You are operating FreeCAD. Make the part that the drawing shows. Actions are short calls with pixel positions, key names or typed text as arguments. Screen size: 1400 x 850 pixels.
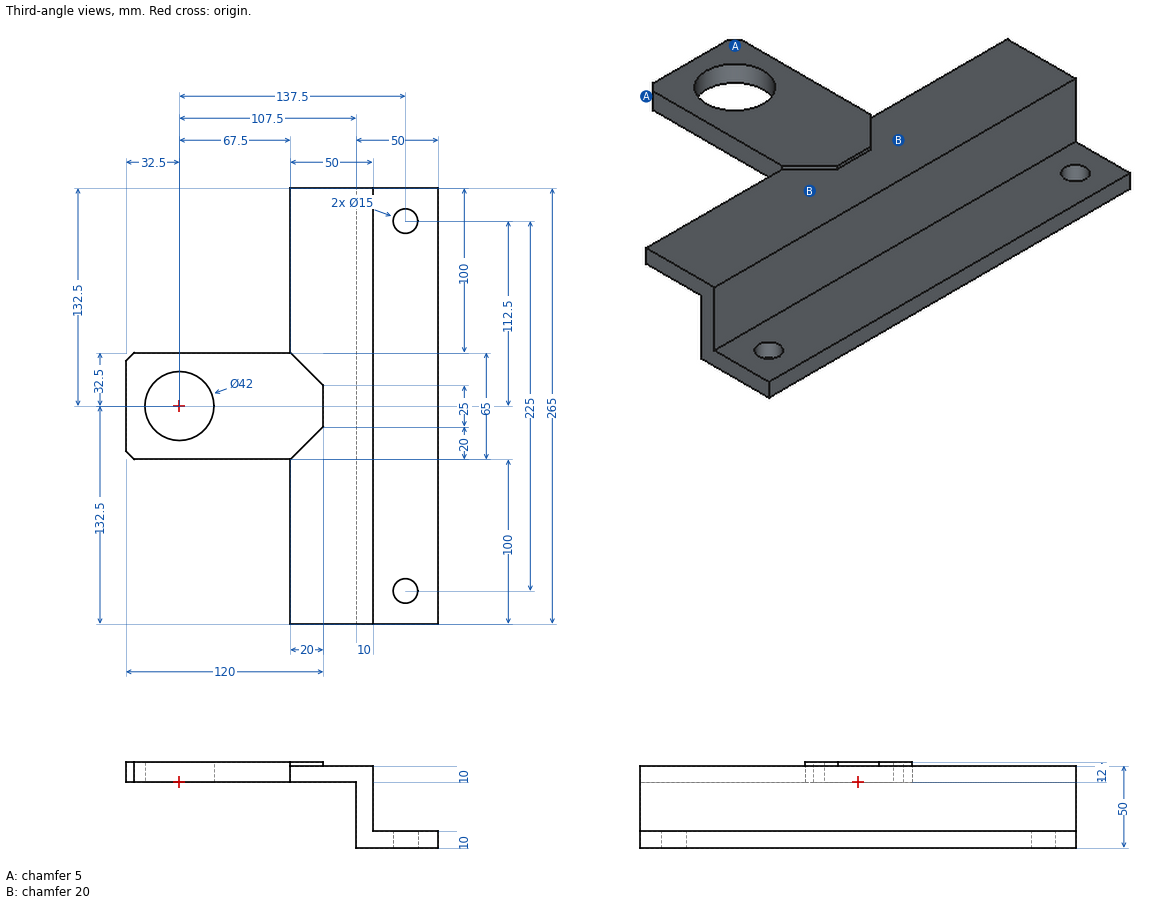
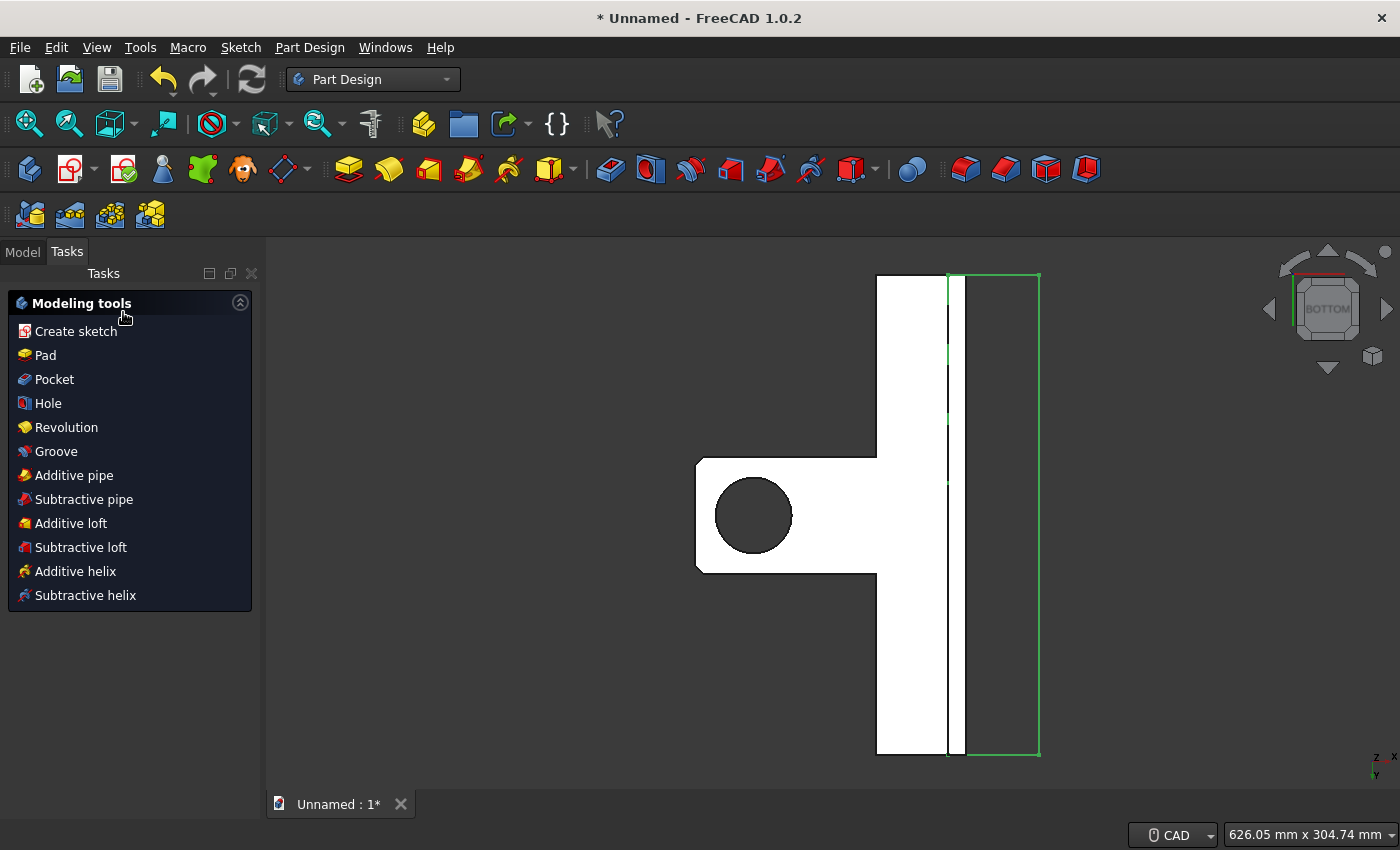
click(350, 170)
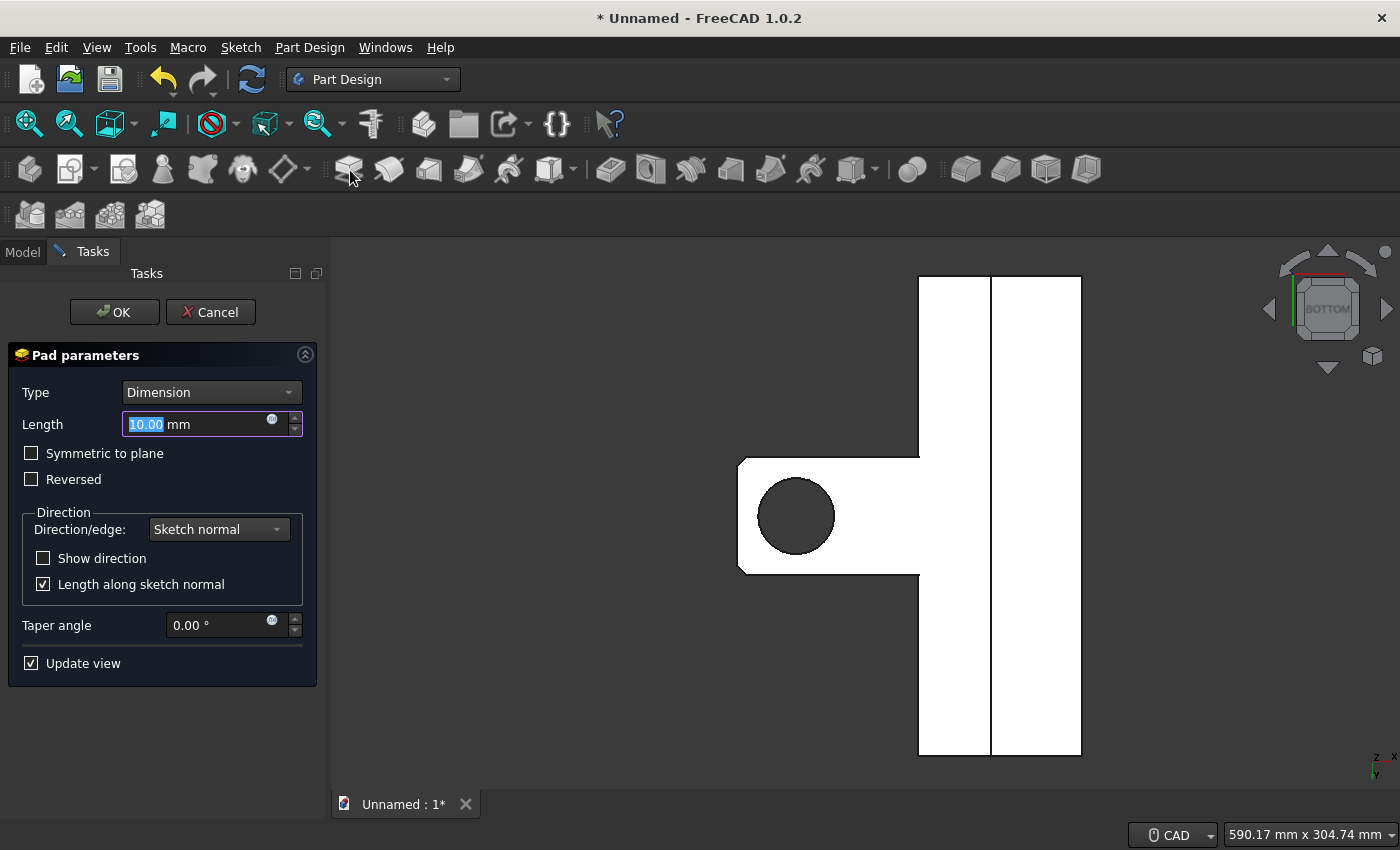
text(10)
key(Tab)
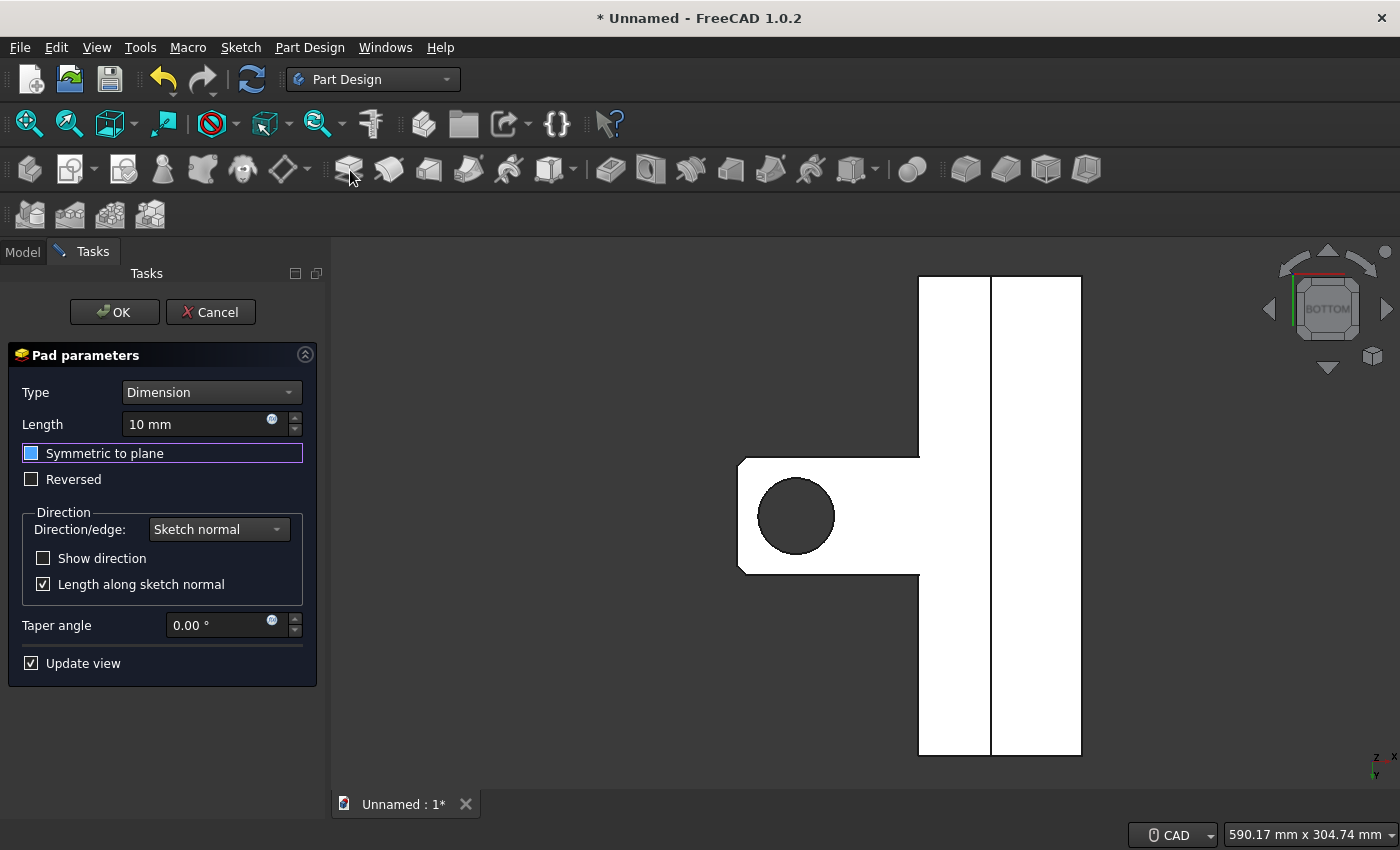
click(30, 479)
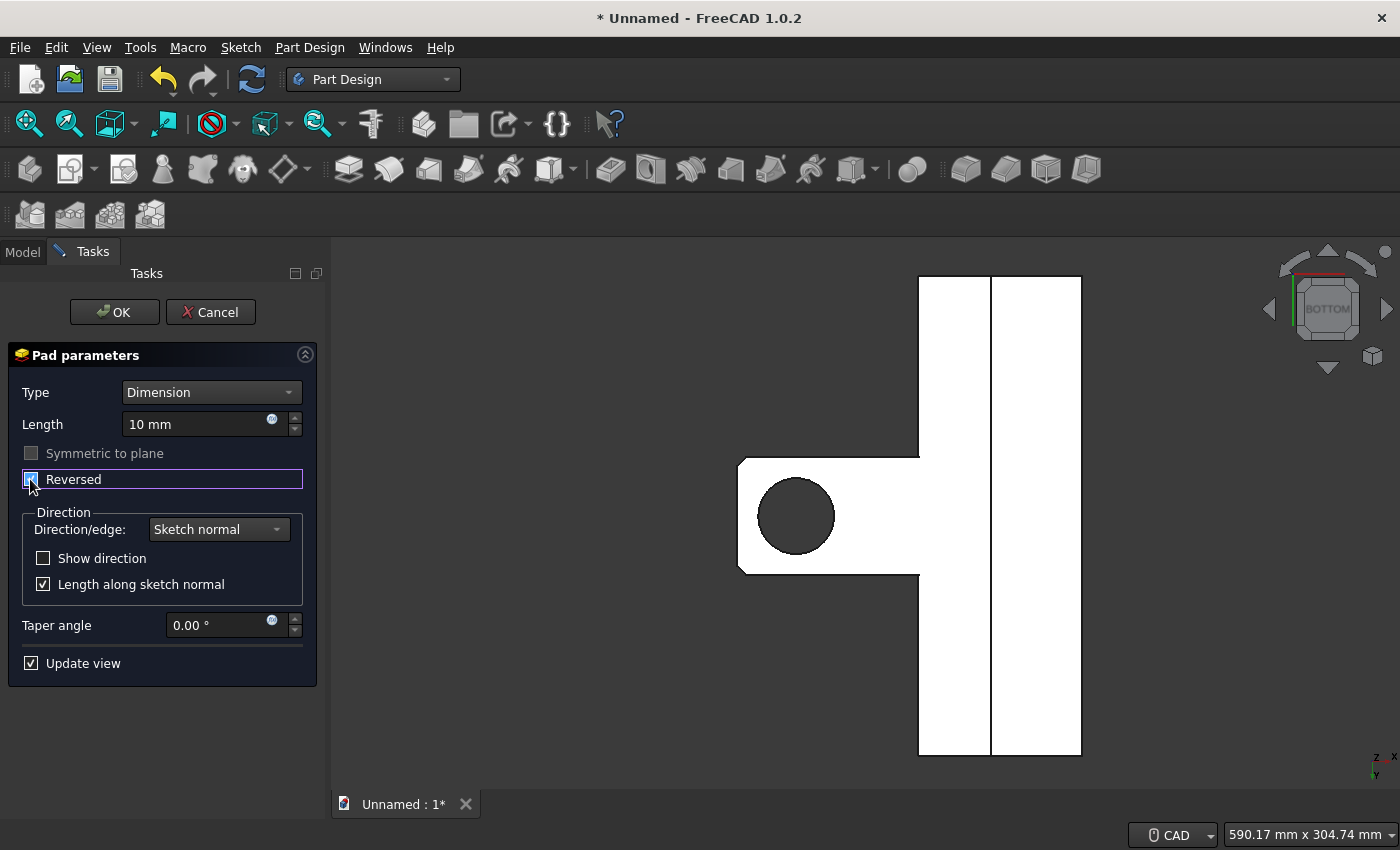
click(115, 312)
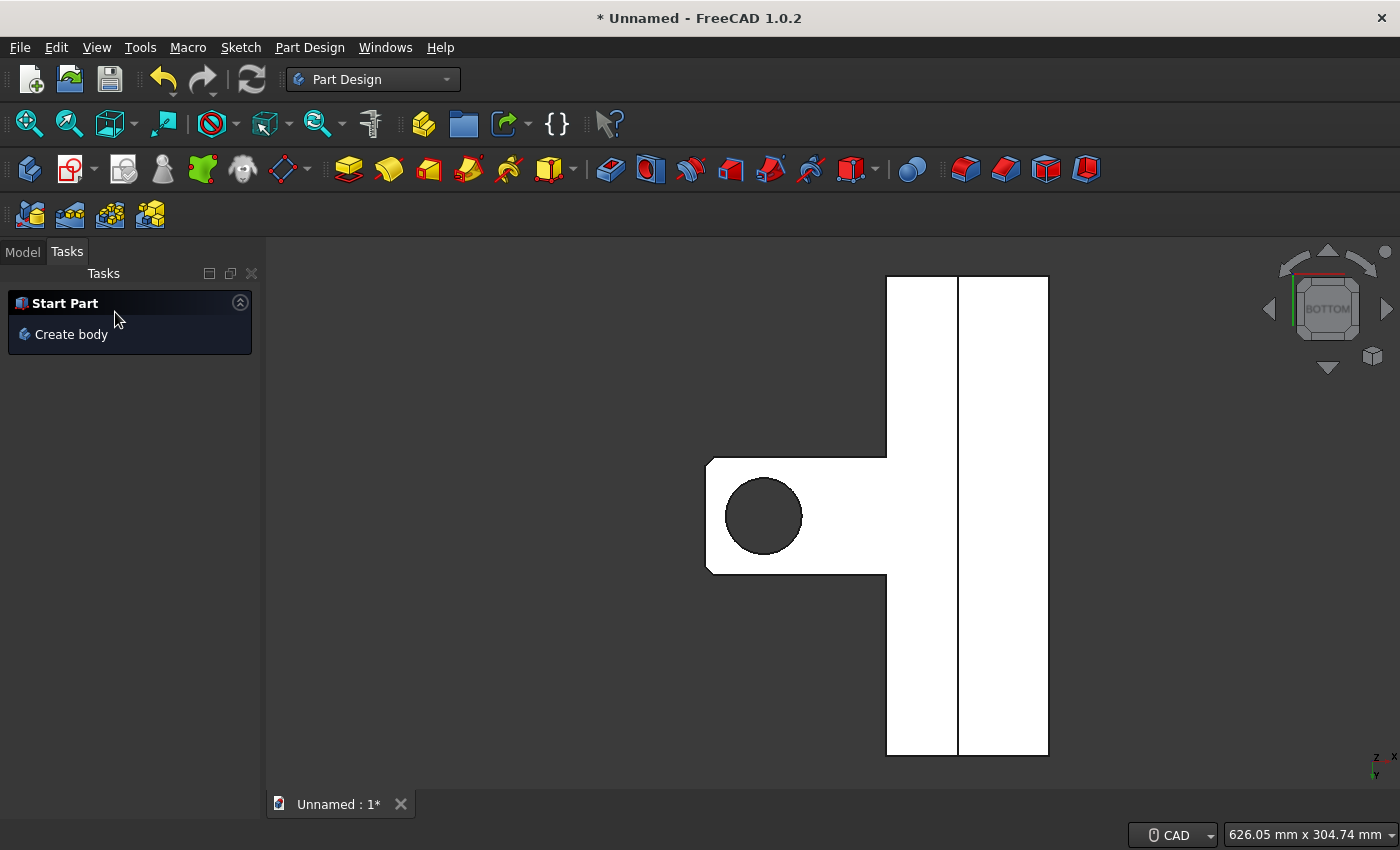
key(0)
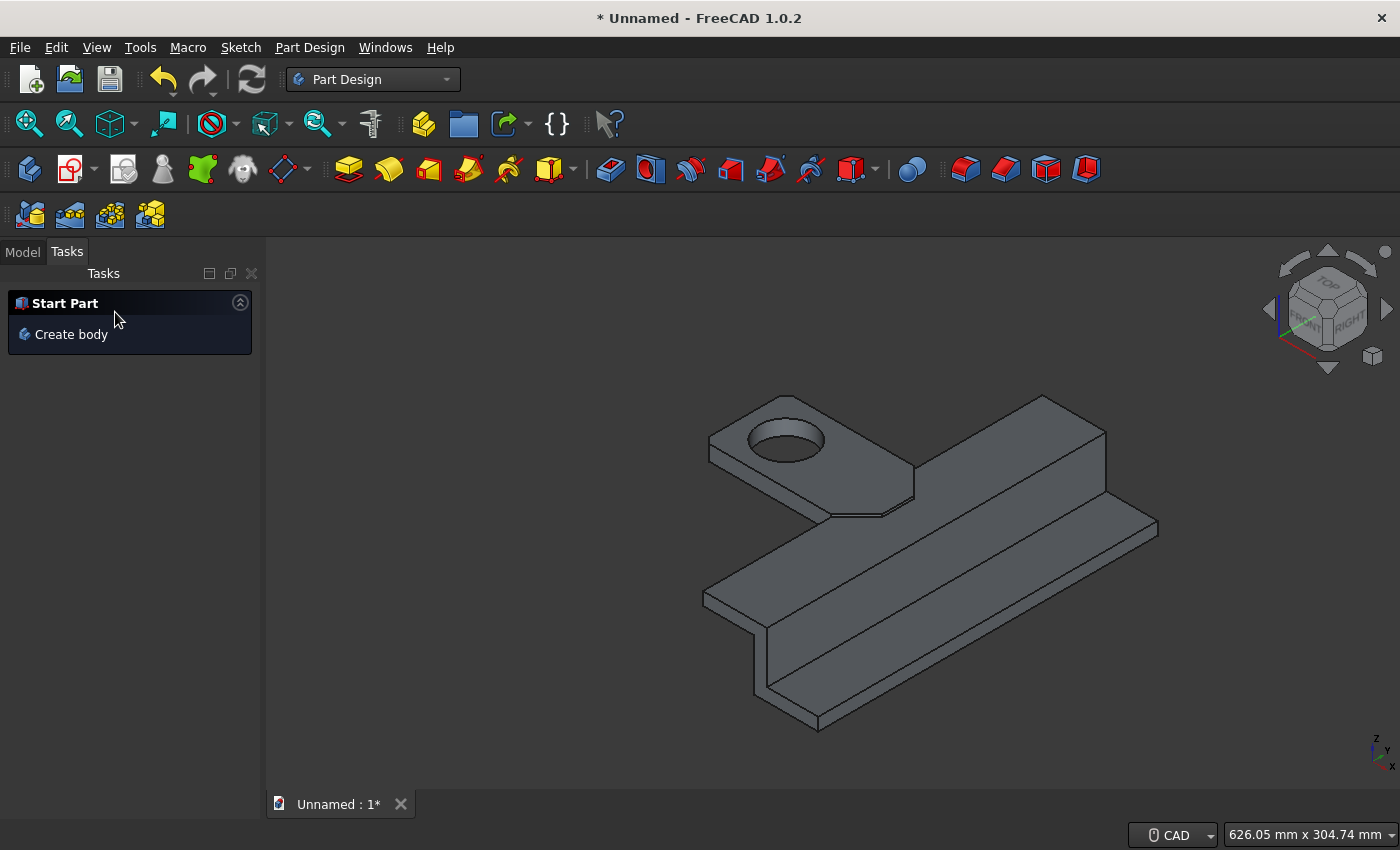
click(1059, 547)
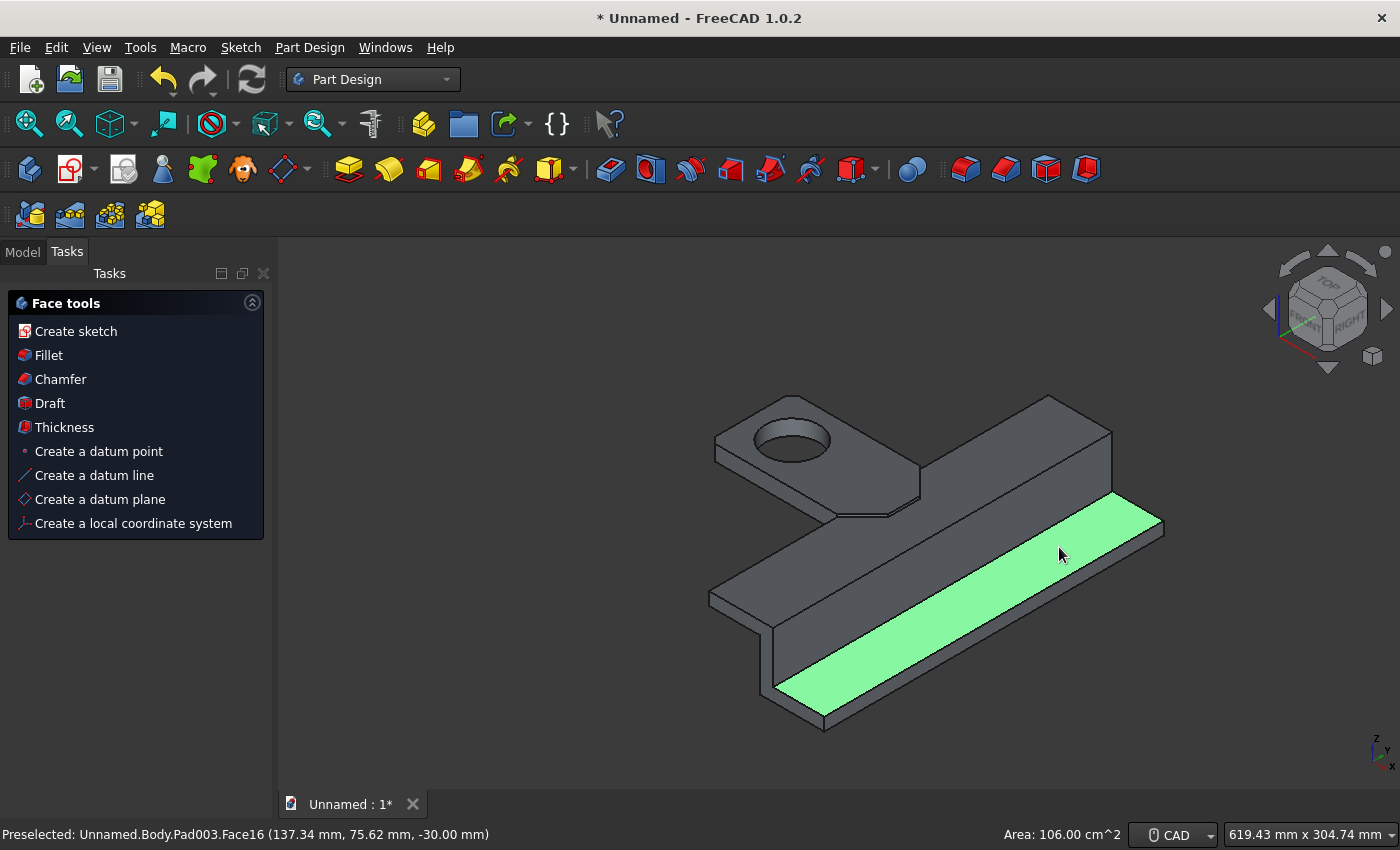
click(70, 170)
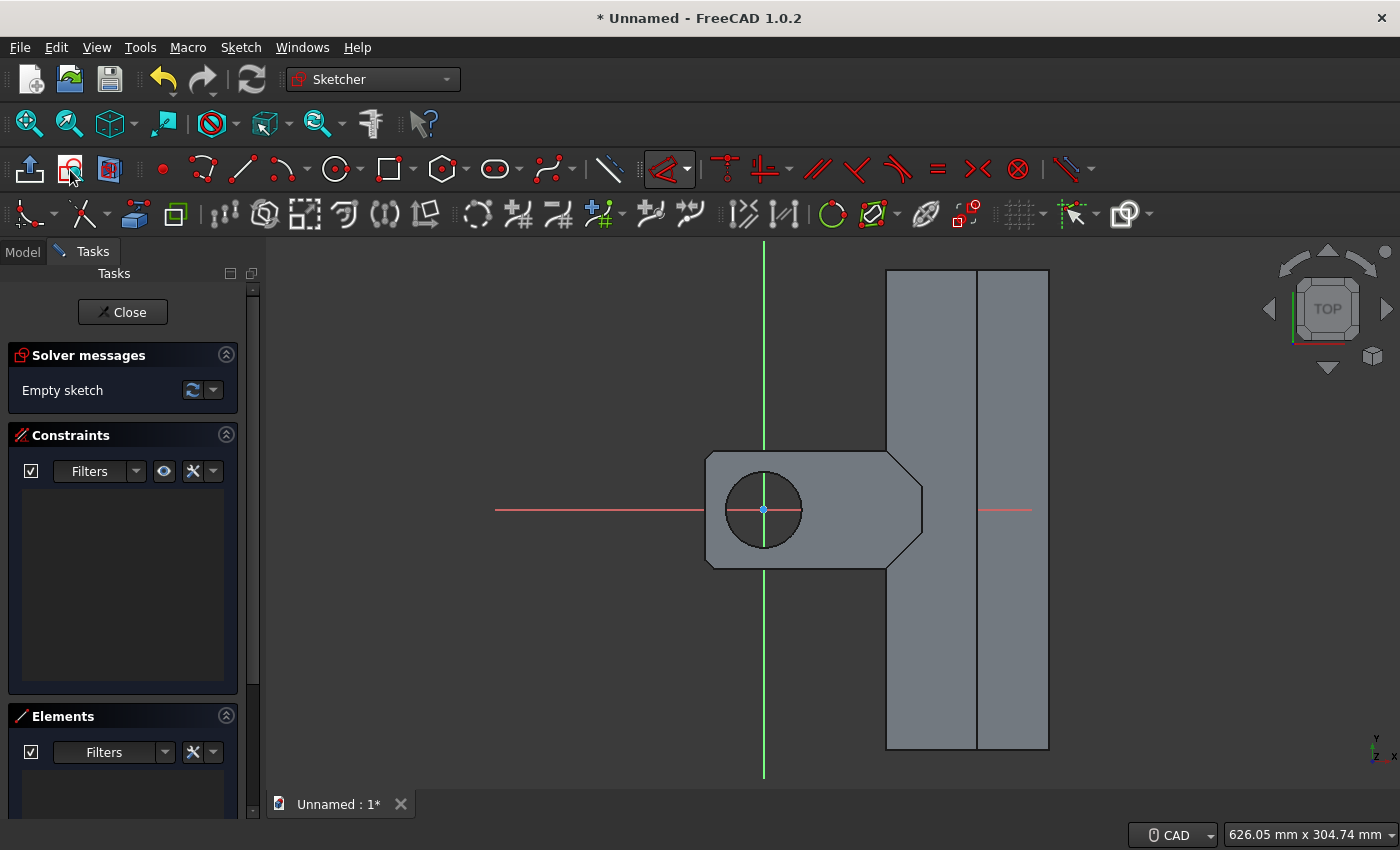
key(g)
key(c)